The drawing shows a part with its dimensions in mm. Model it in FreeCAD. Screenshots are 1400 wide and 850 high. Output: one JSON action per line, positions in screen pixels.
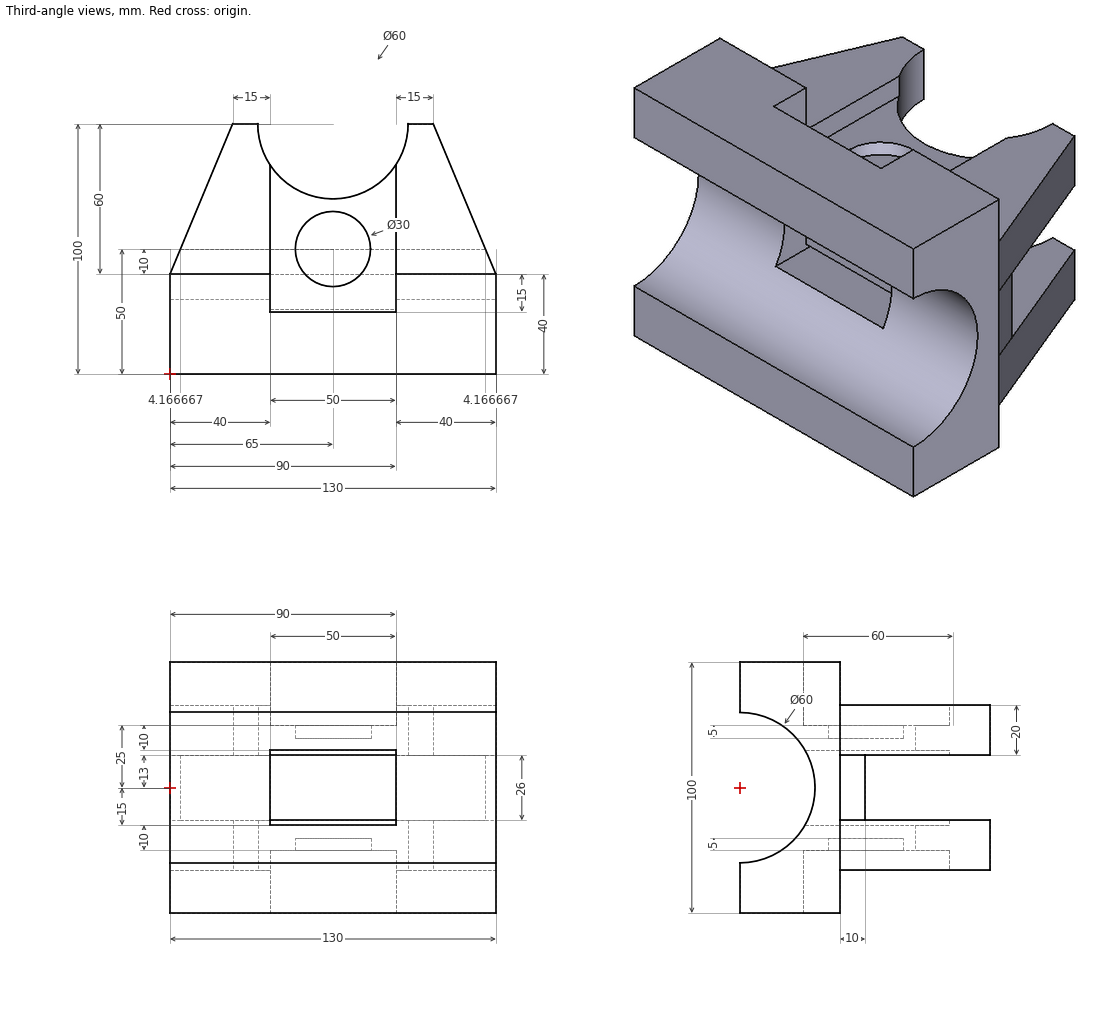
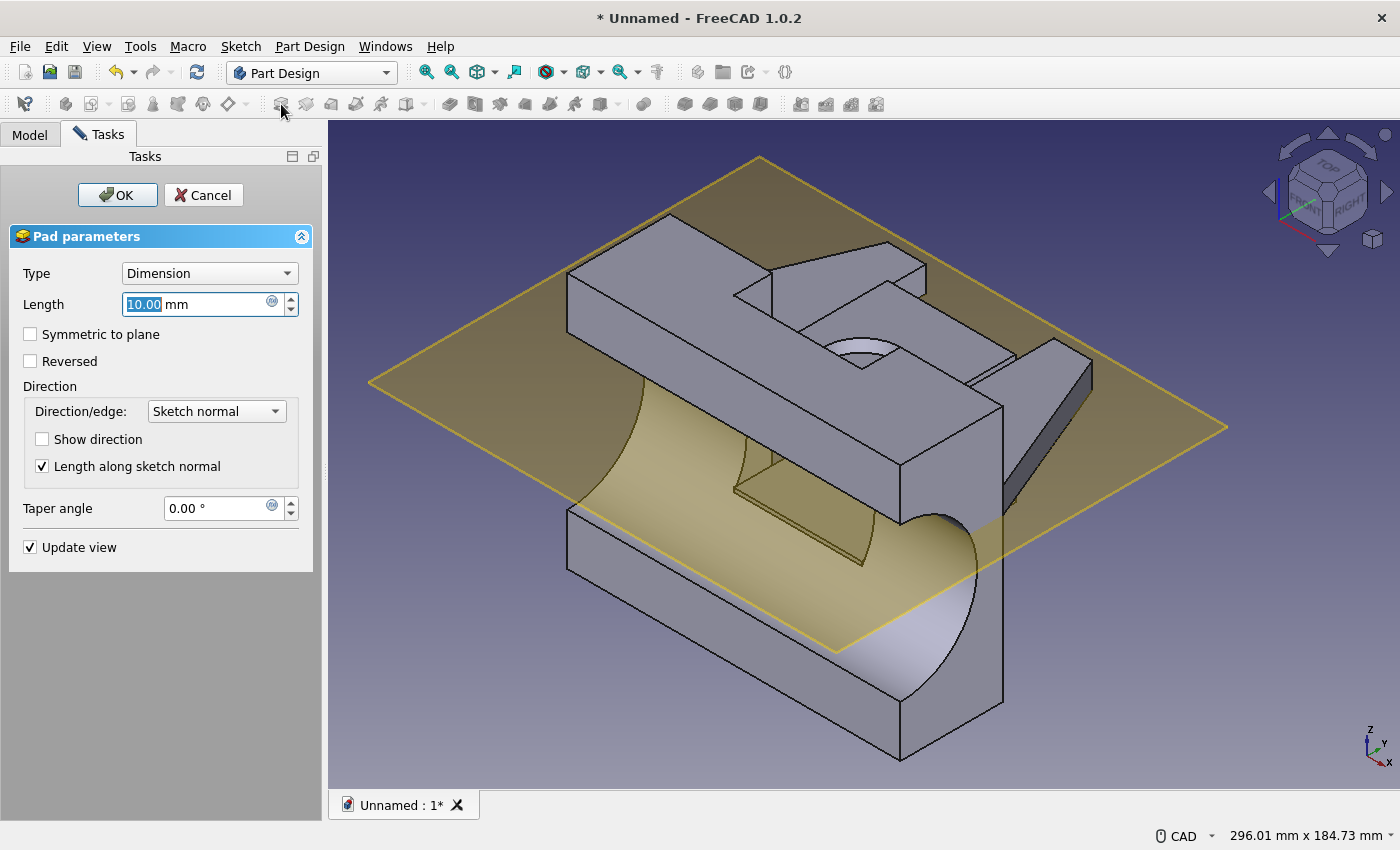
{"action": "type", "text": "20"}
{"action": "key", "text": "Tab"}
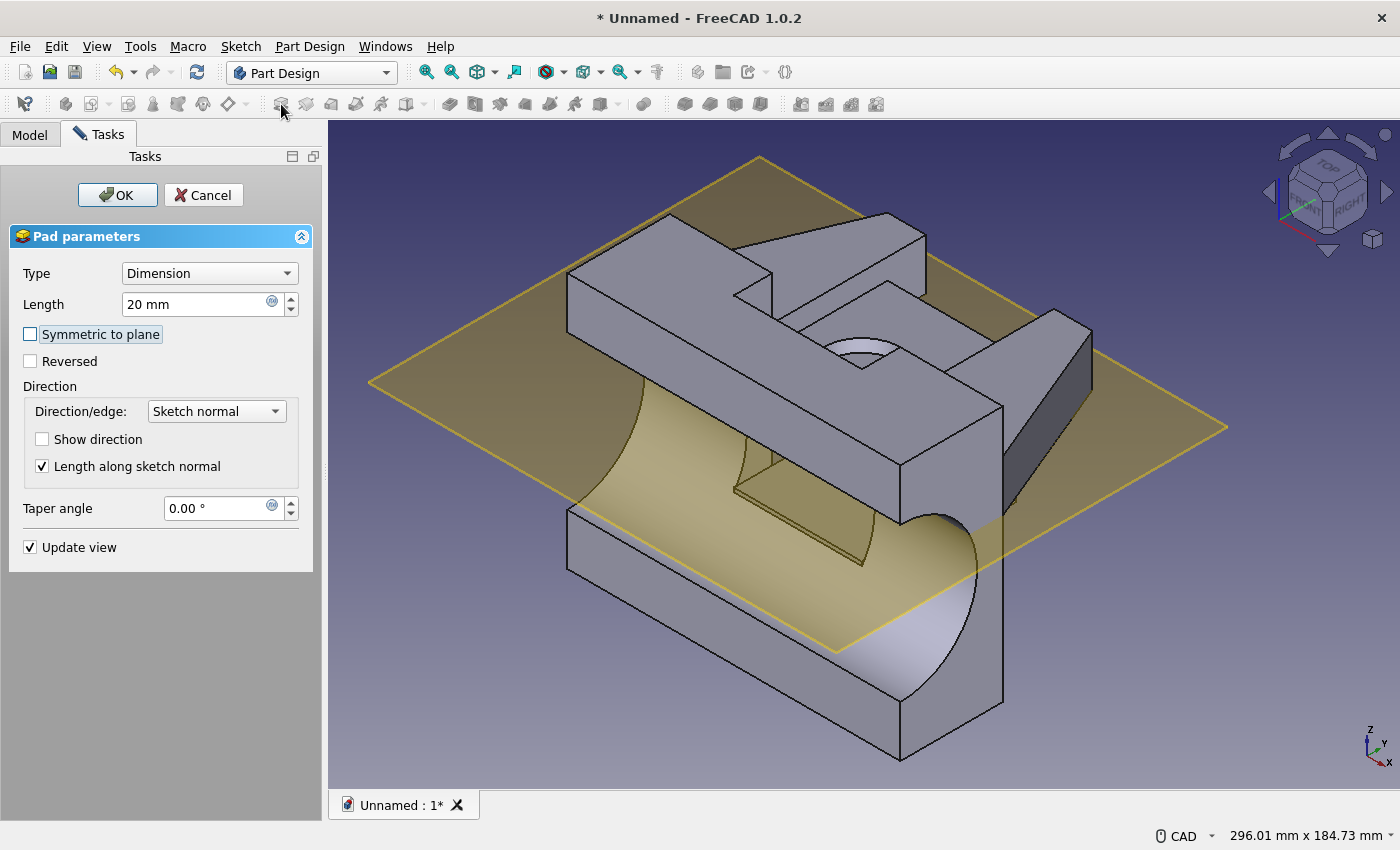
{"action": "left_click", "coordinate": [118, 195]}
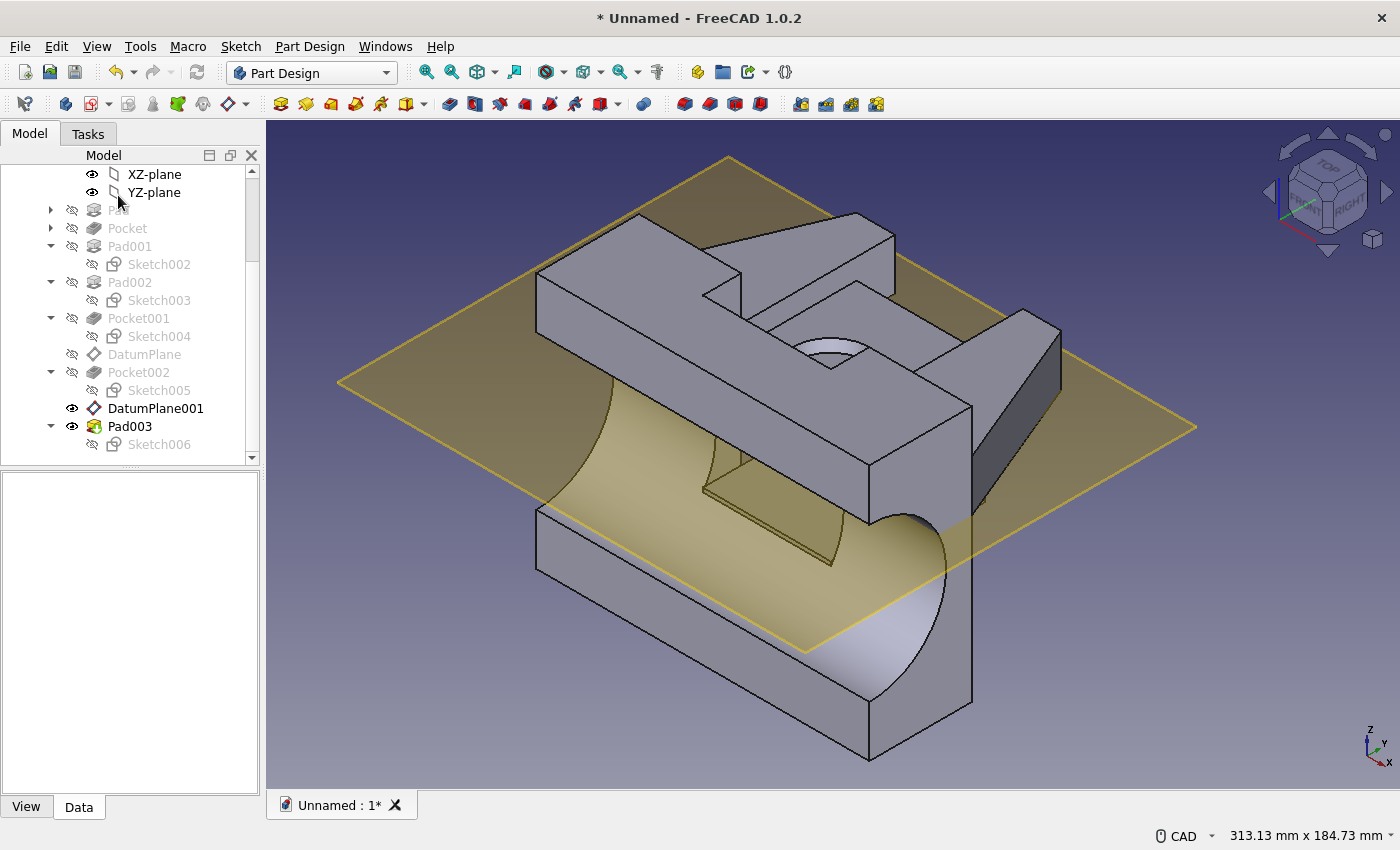
{"action": "left_click", "coordinate": [117, 408]}
{"action": "key", "text": "space"}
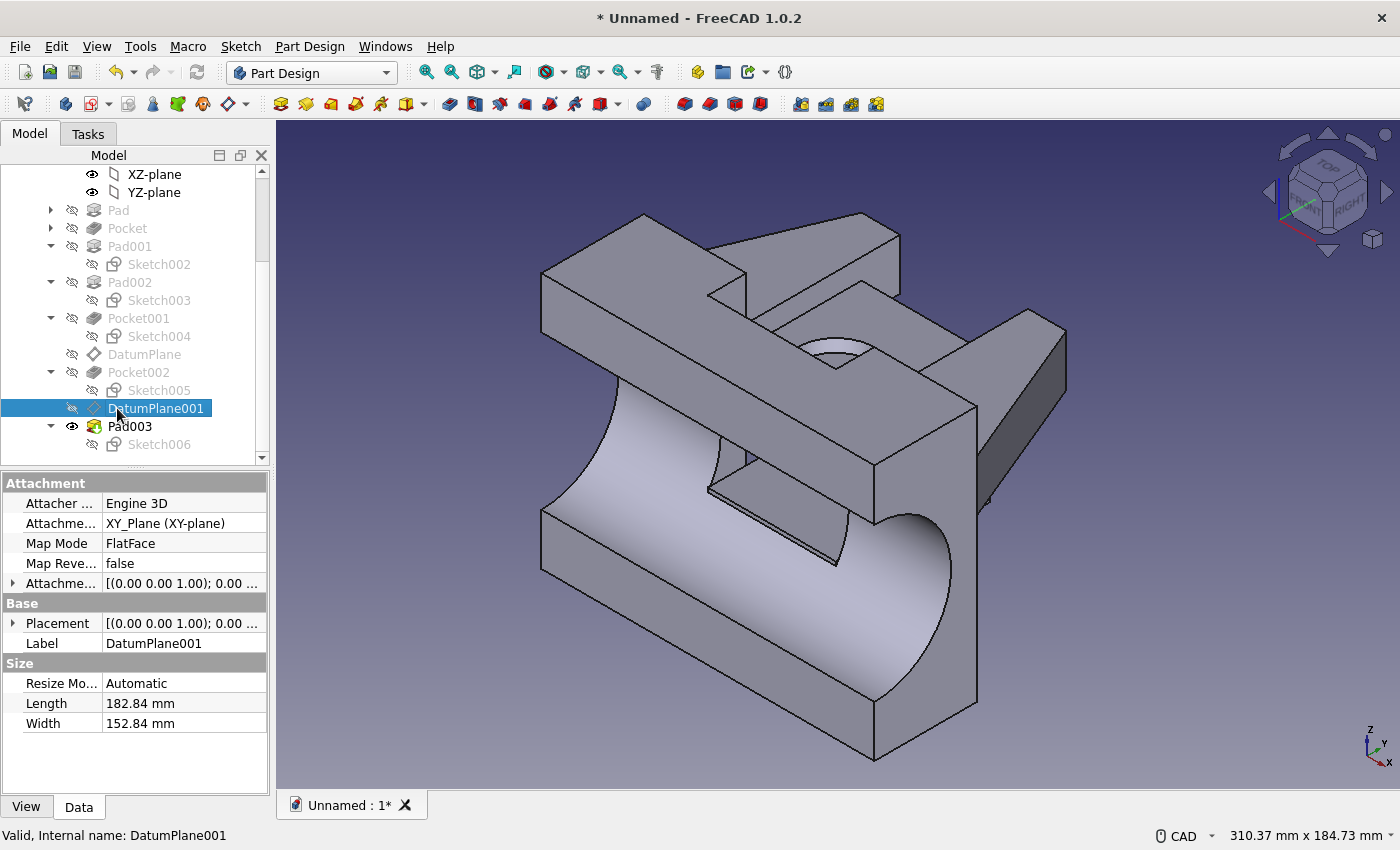
{"action": "key", "text": "5"}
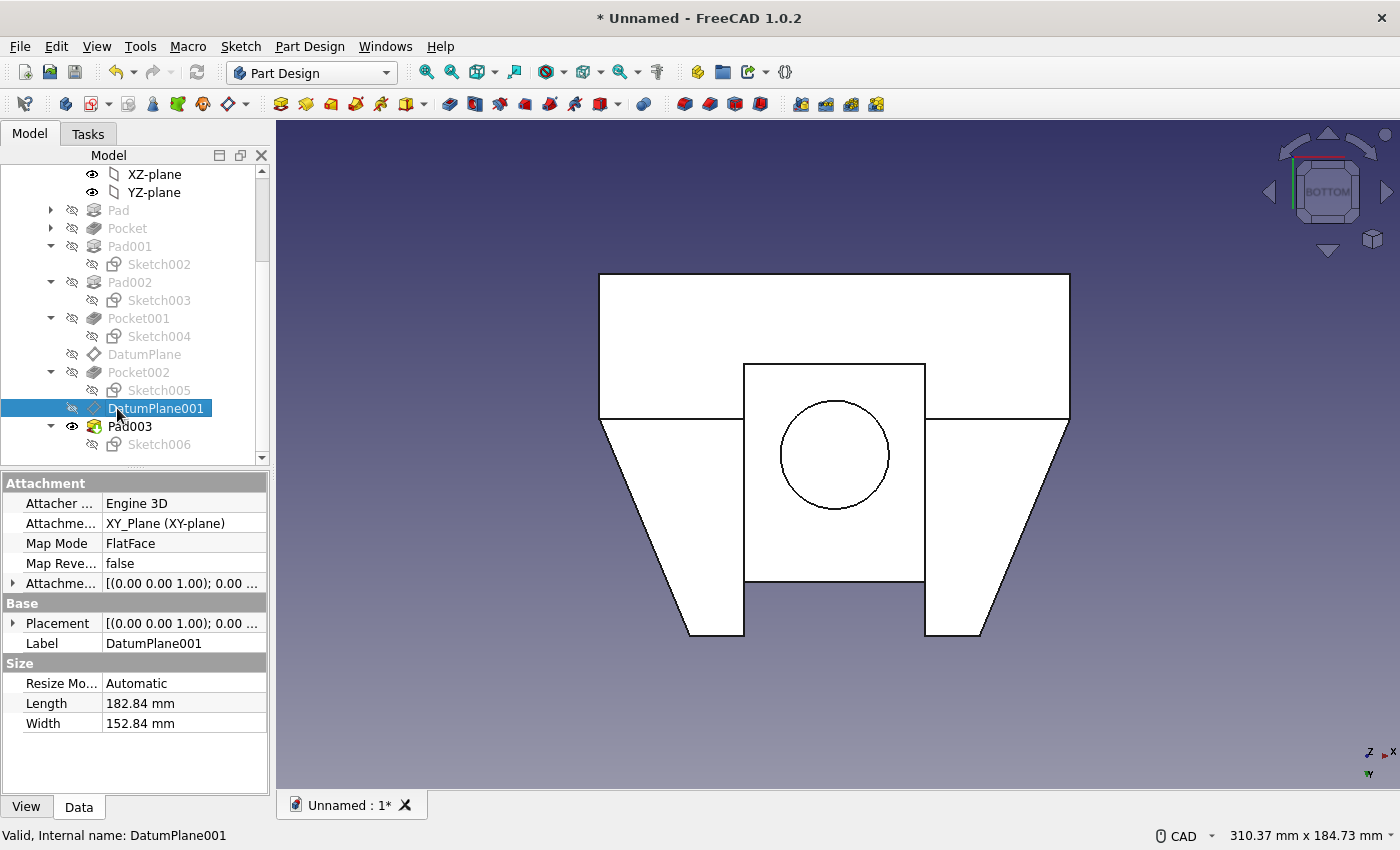
{"action": "left_click", "coordinate": [977, 495]}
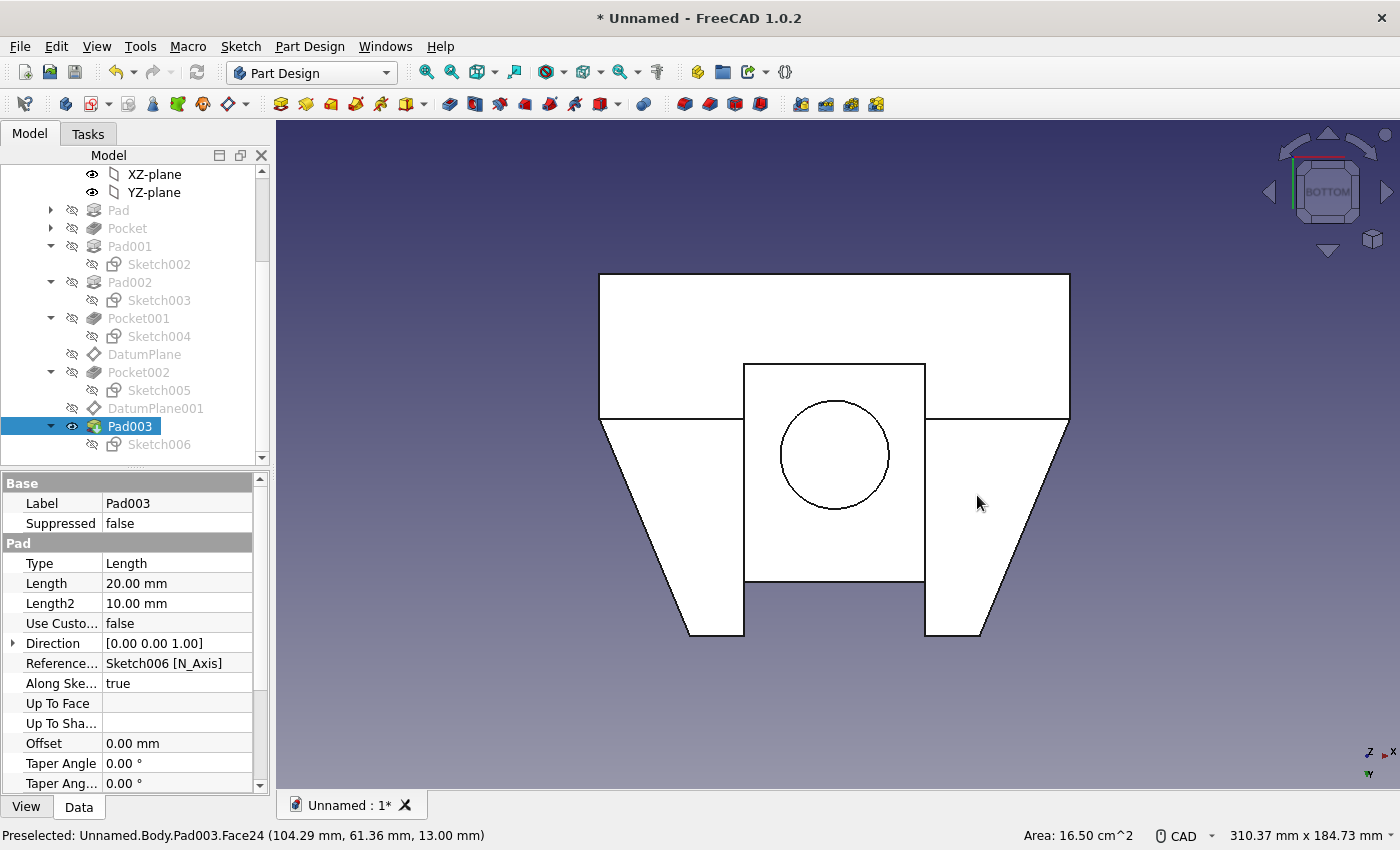
{"action": "left_click", "coordinate": [90, 104]}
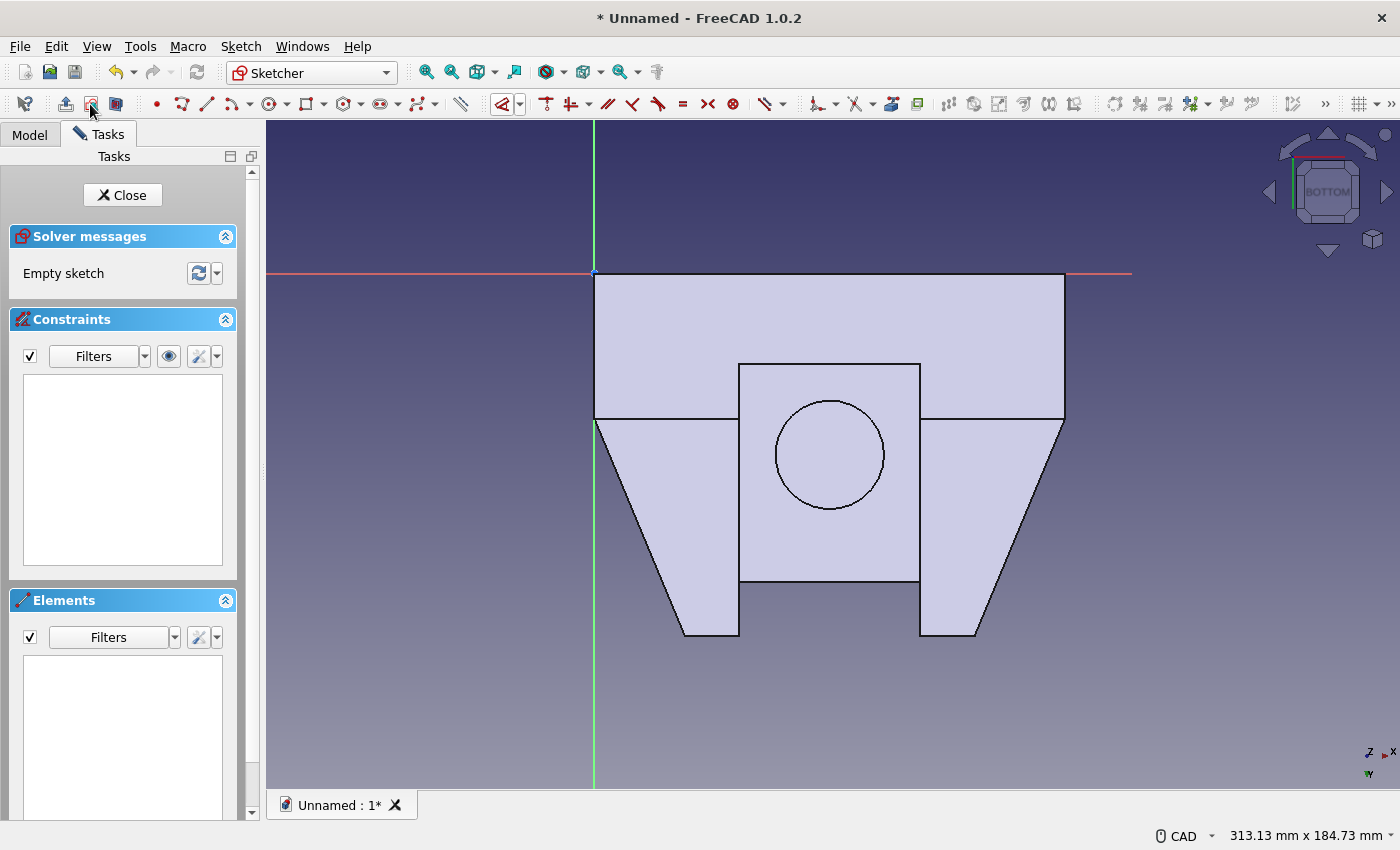
{"action": "left_click", "coordinate": [116, 104]}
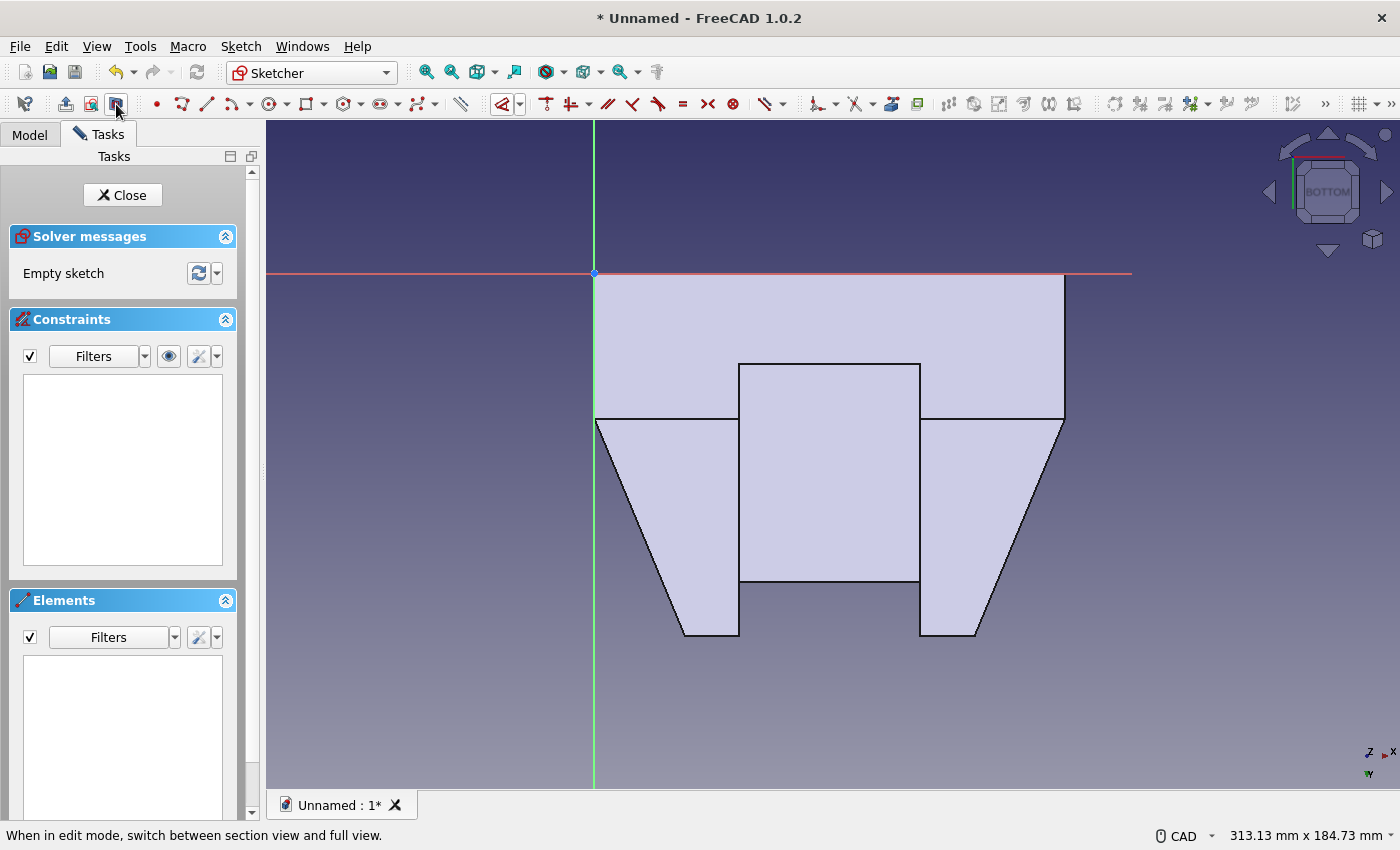
{"action": "scroll", "coordinate": [756, 208], "scroll_direction": "down", "scroll_amount": 1}